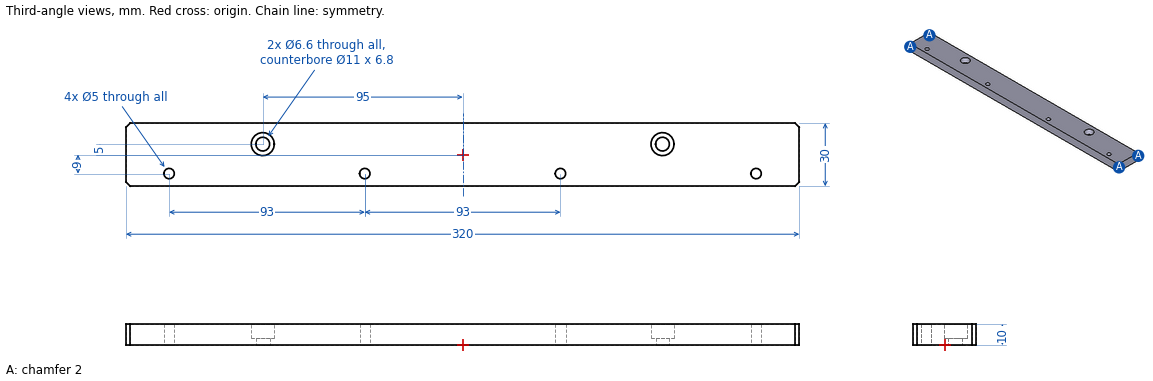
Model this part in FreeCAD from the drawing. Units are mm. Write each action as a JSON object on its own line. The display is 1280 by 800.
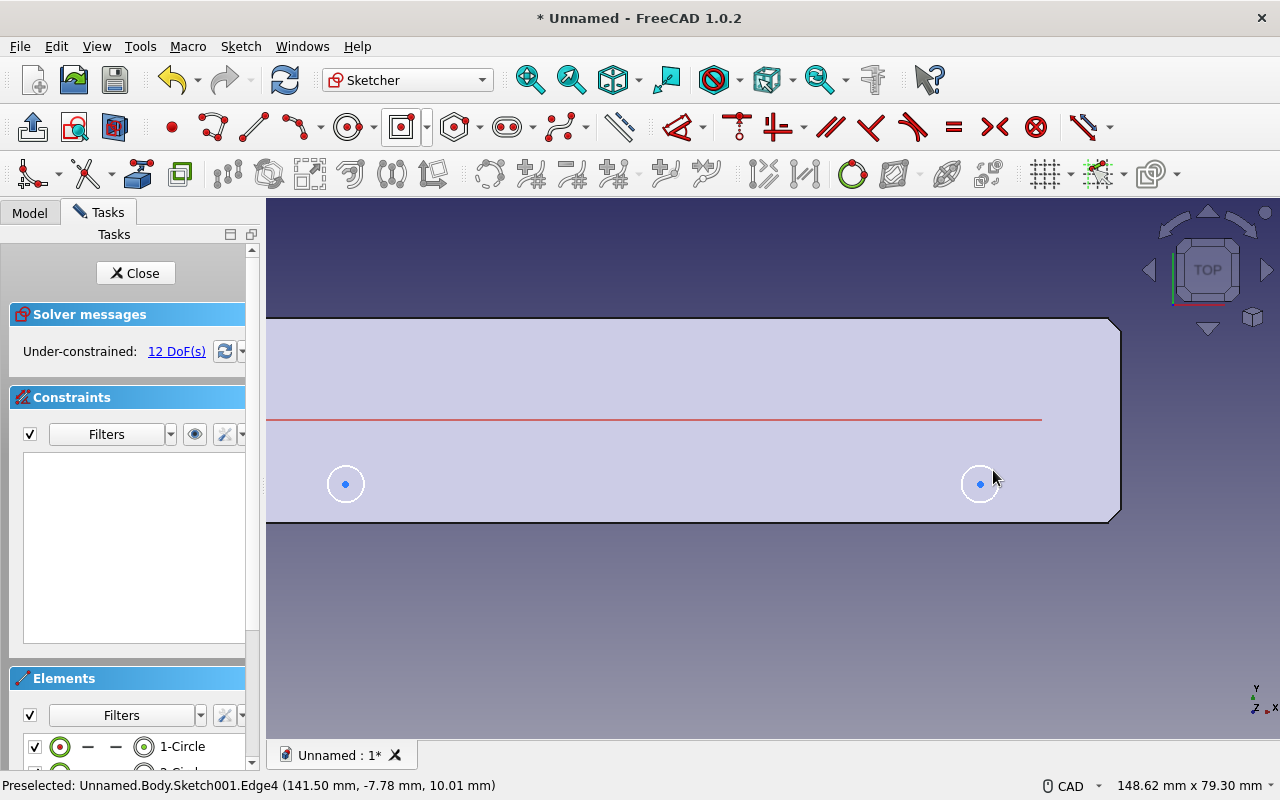
{"action": "scroll", "coordinate": [995, 472], "scroll_direction": "down", "scroll_amount": 6}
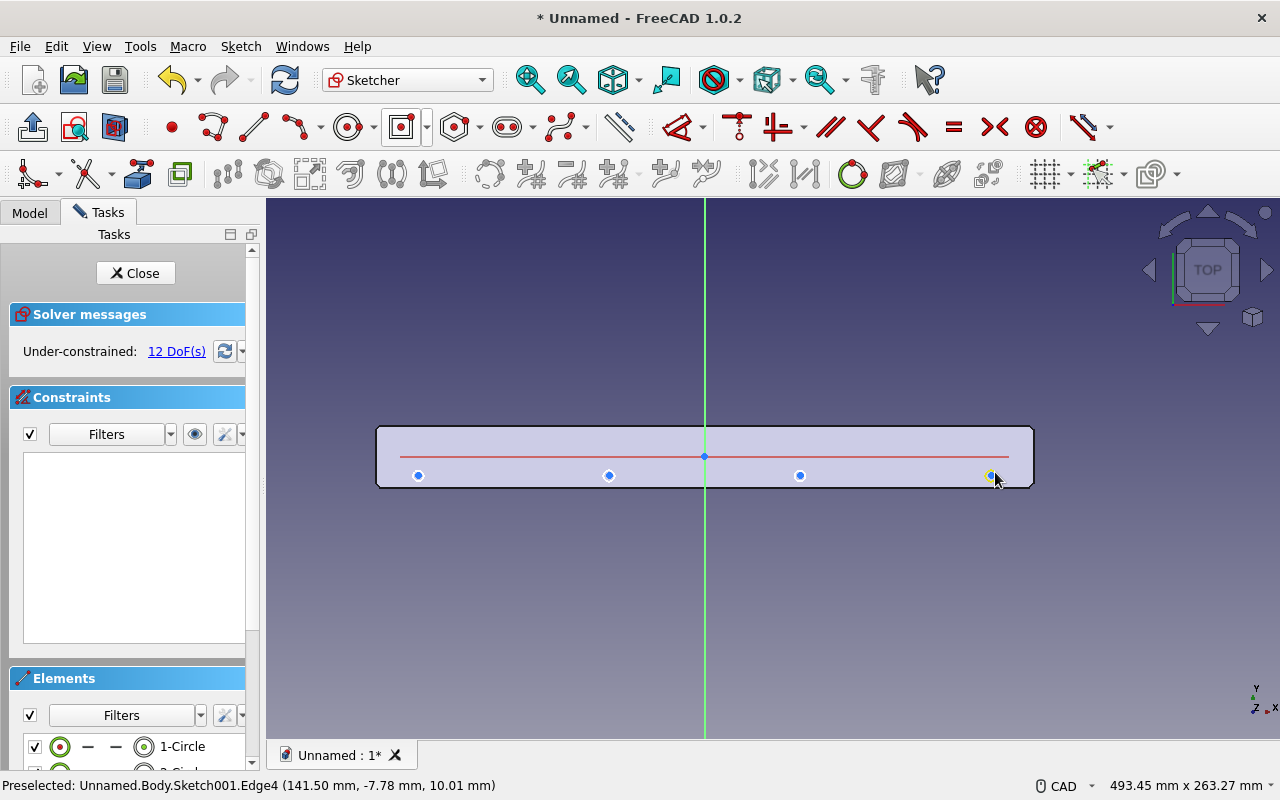
{"action": "scroll", "coordinate": [422, 472], "scroll_direction": "up", "scroll_amount": 5}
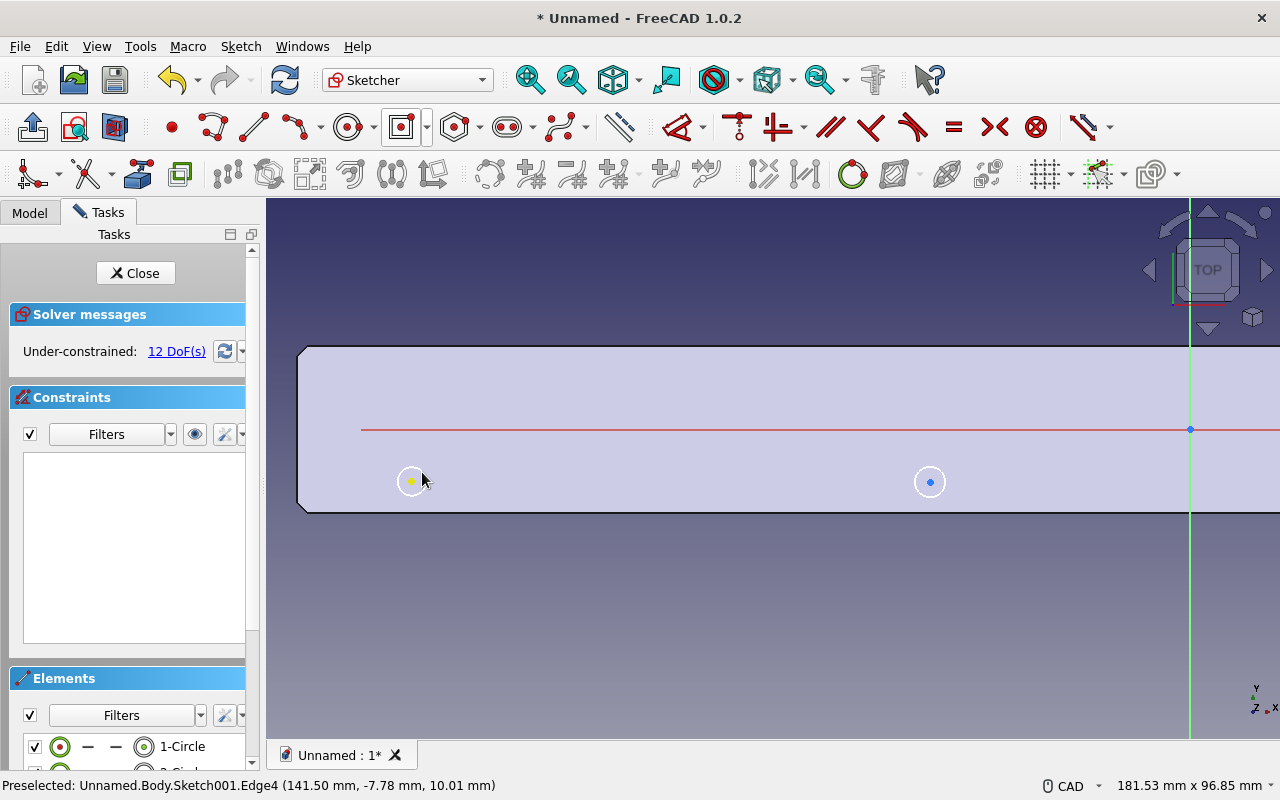
{"action": "left_click", "coordinate": [422, 471]}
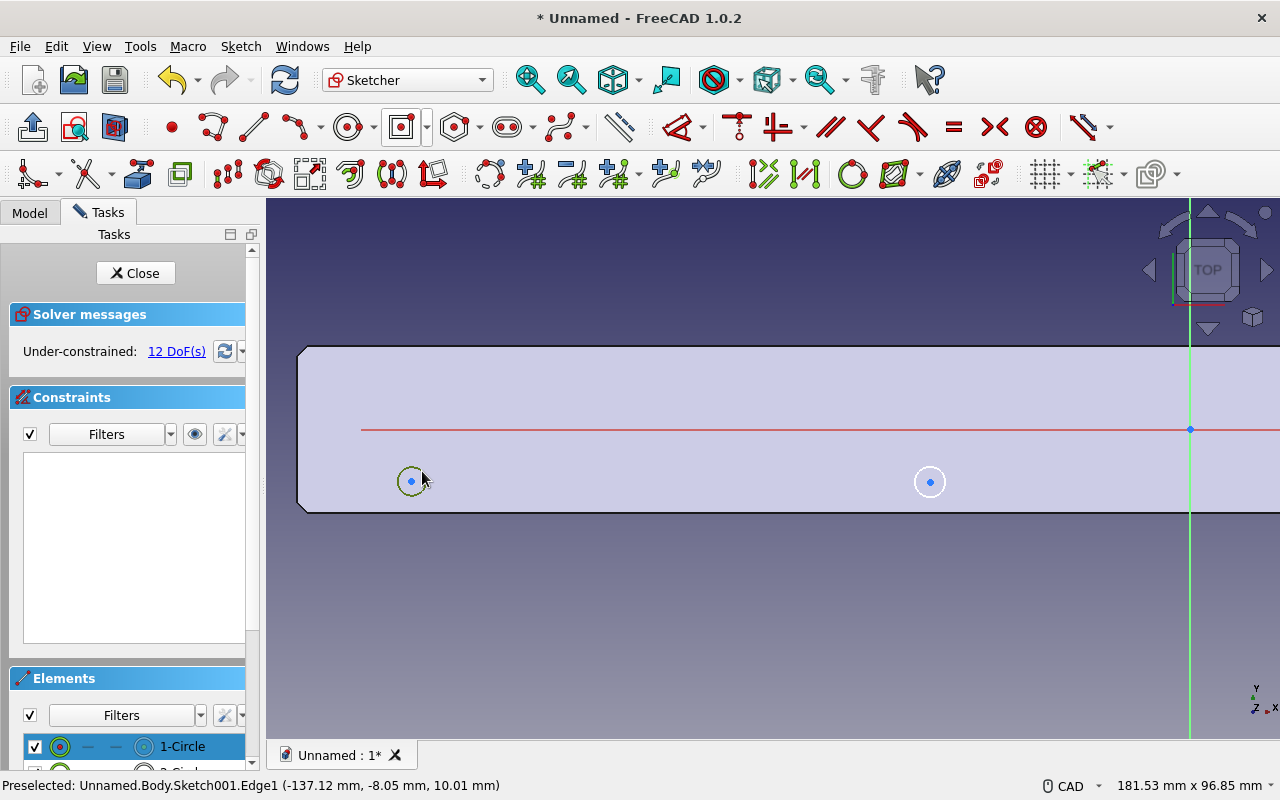
{"action": "left_click", "coordinate": [941, 471]}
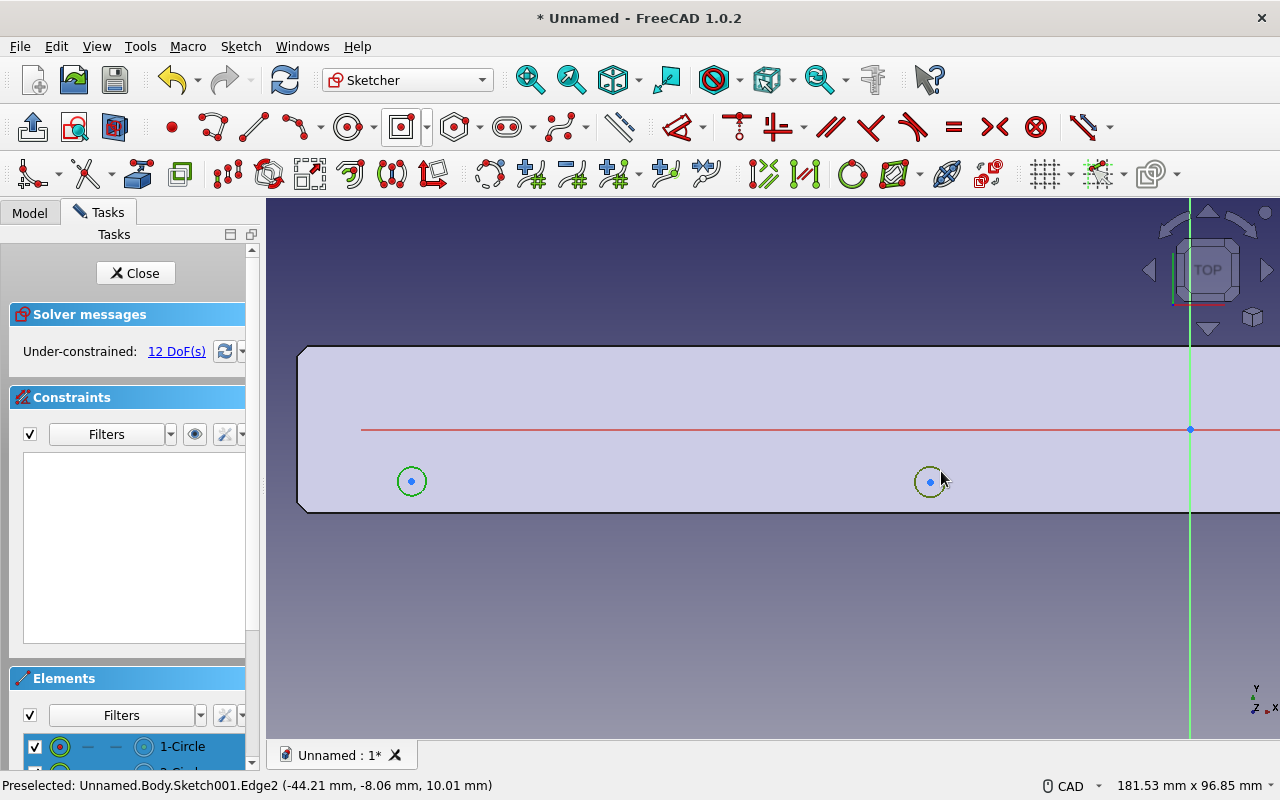
{"action": "scroll", "coordinate": [422, 472], "scroll_direction": "down", "scroll_amount": 5}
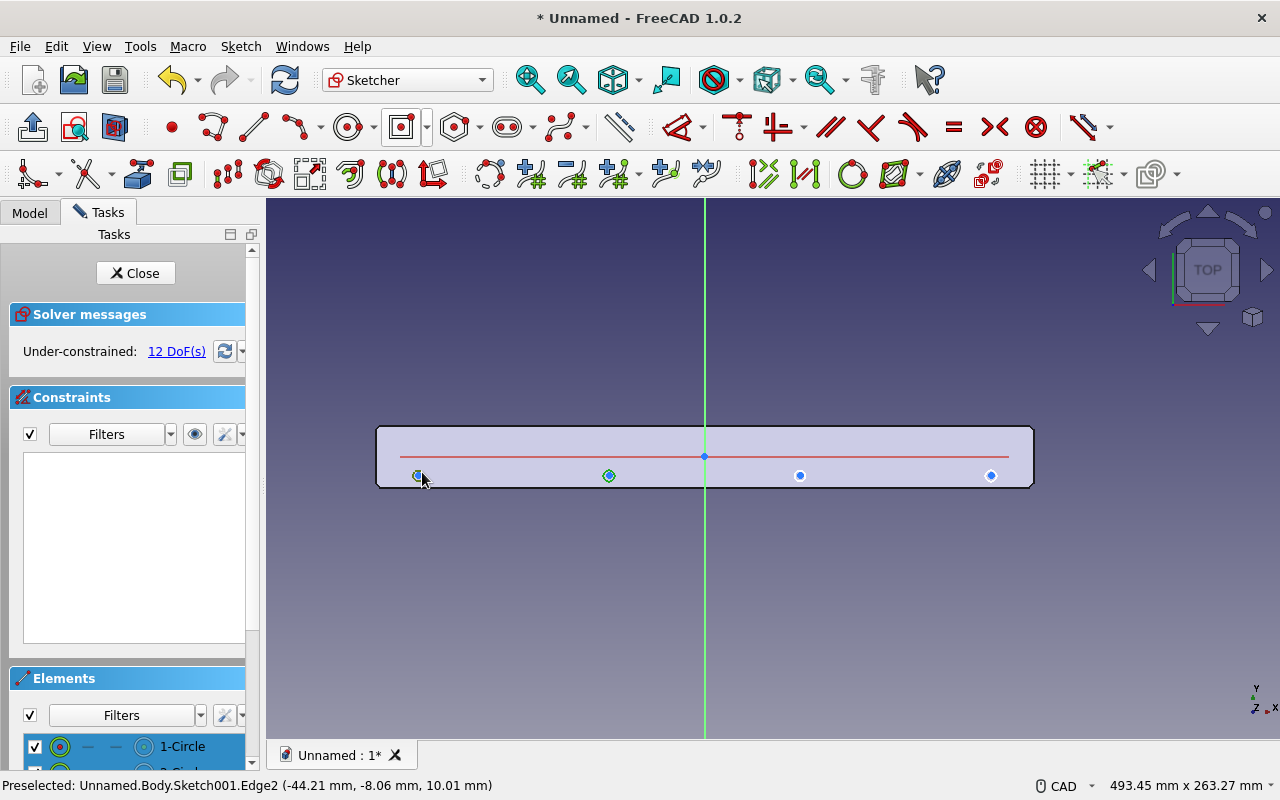
{"action": "scroll", "coordinate": [804, 472], "scroll_direction": "up", "scroll_amount": 5}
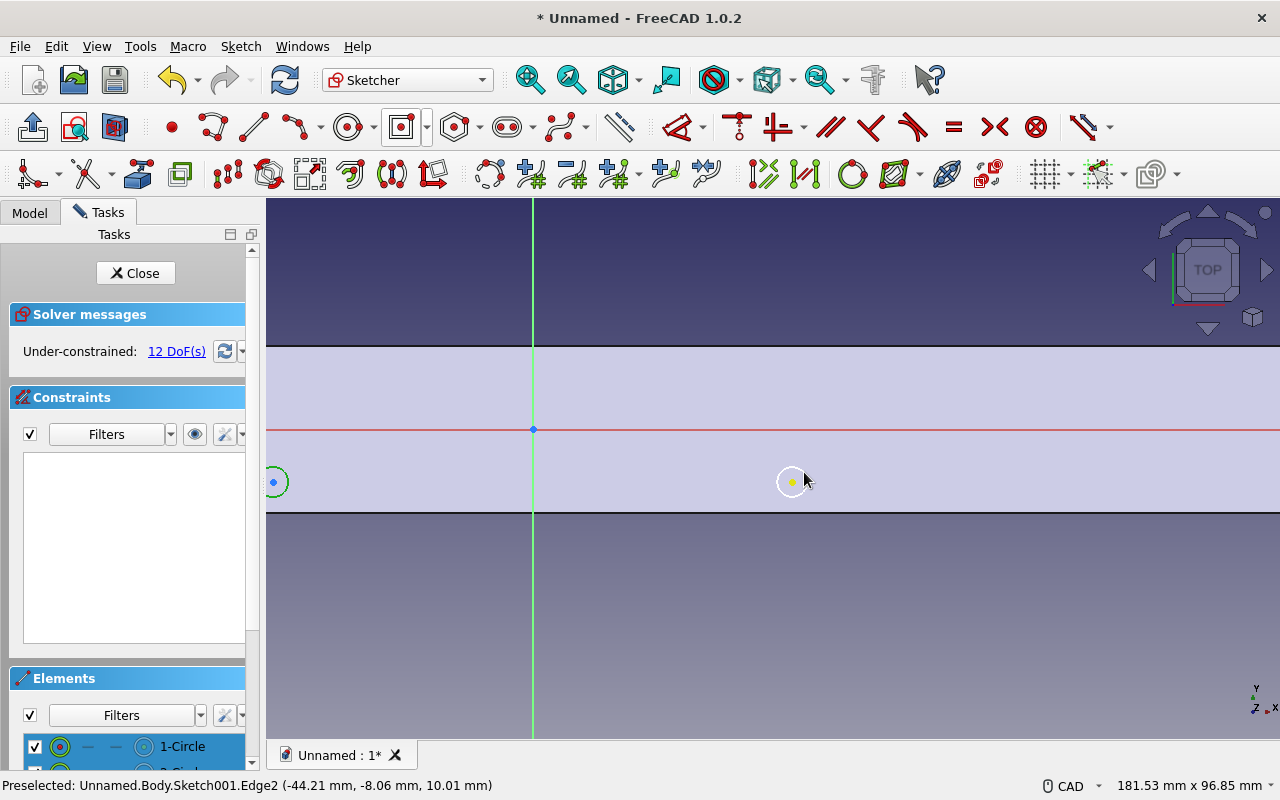
{"action": "left_click", "coordinate": [803, 471]}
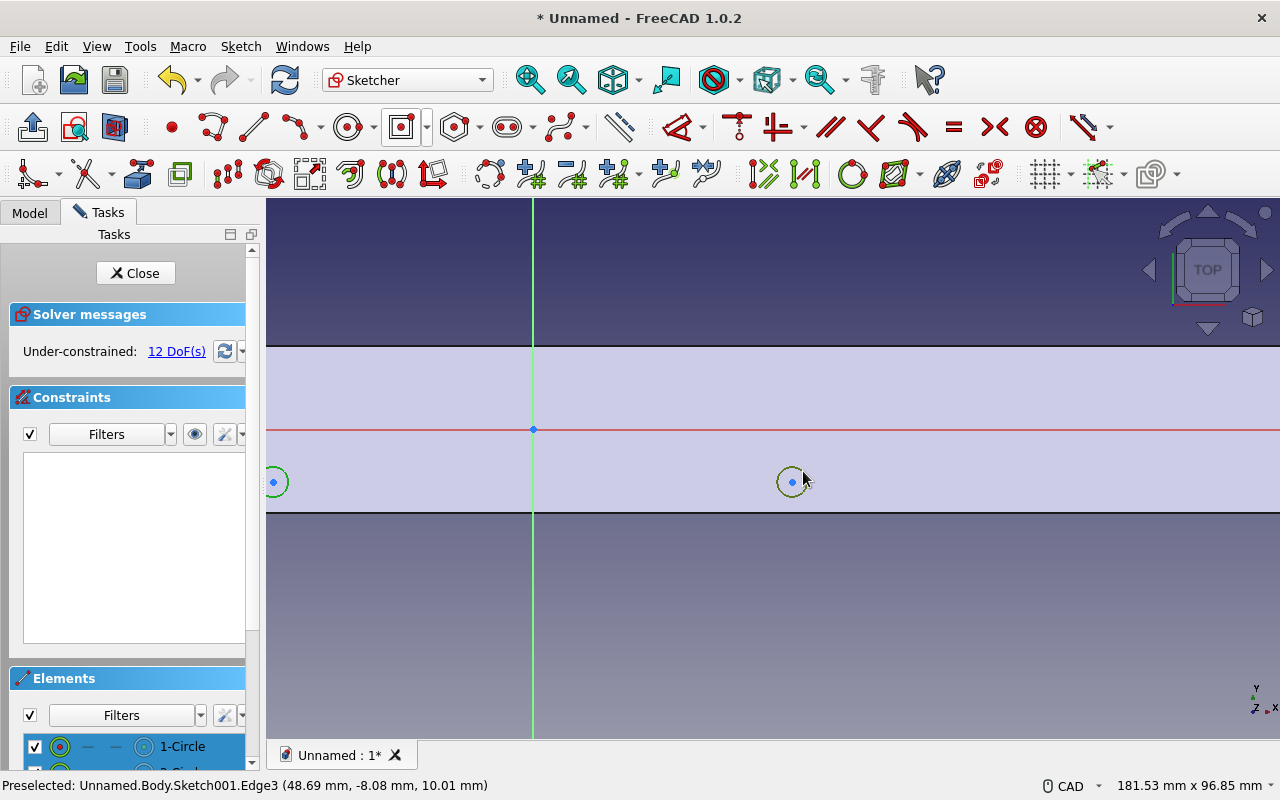
{"action": "scroll", "coordinate": [804, 472], "scroll_direction": "down", "scroll_amount": 5}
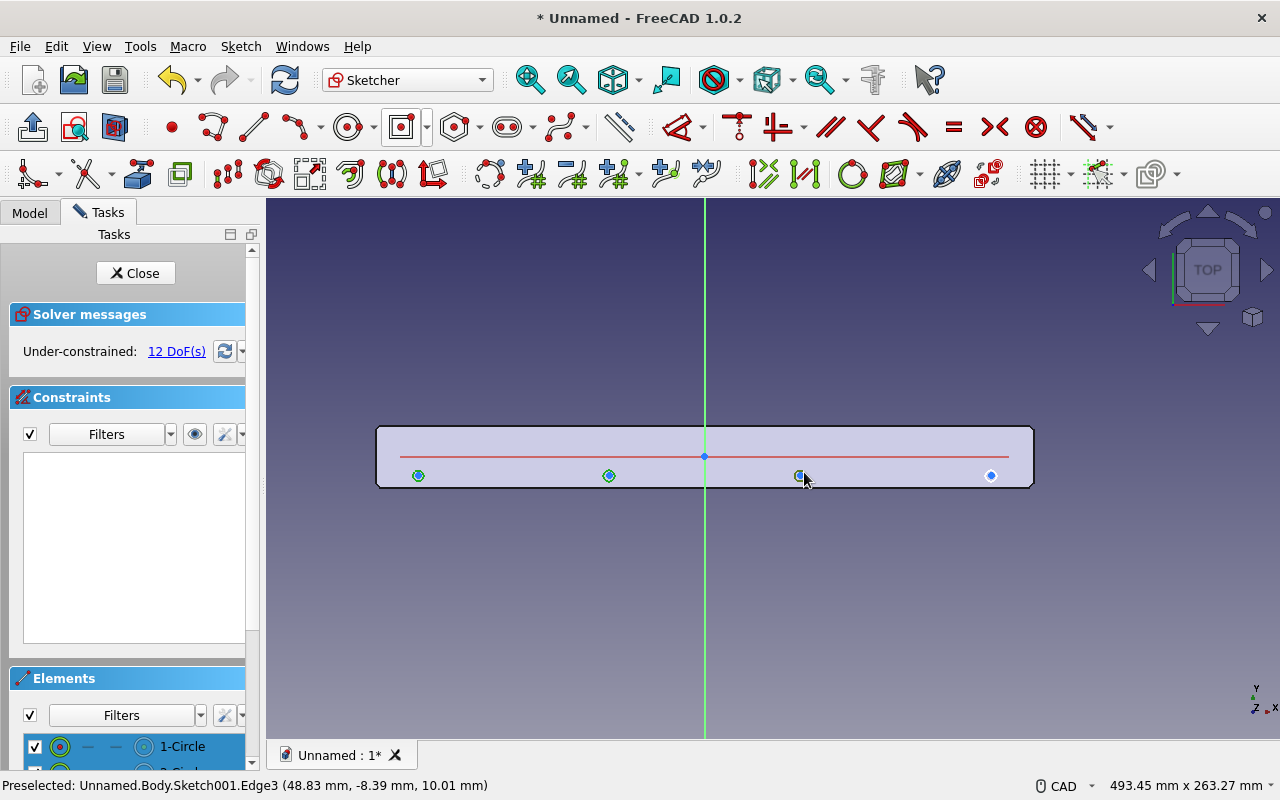
{"action": "scroll", "coordinate": [995, 472], "scroll_direction": "up", "scroll_amount": 5}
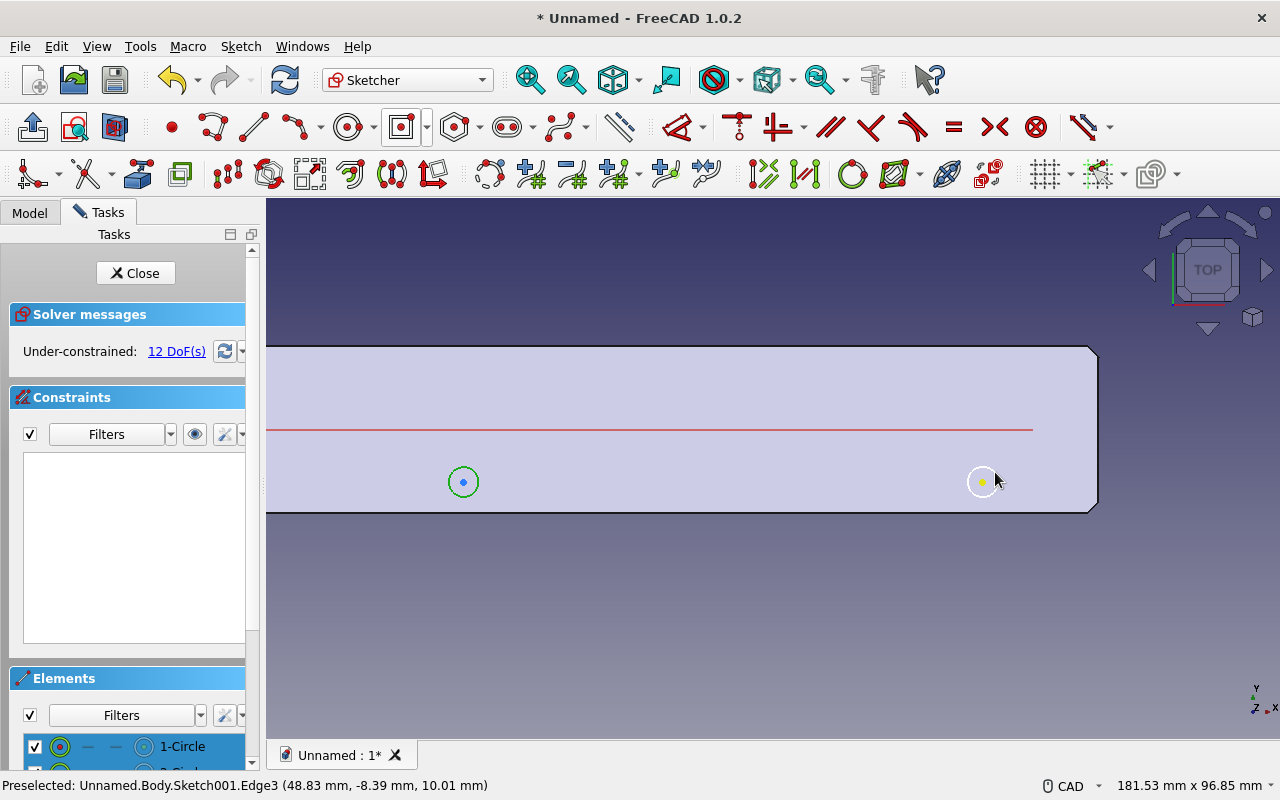
{"action": "left_click", "coordinate": [994, 471]}